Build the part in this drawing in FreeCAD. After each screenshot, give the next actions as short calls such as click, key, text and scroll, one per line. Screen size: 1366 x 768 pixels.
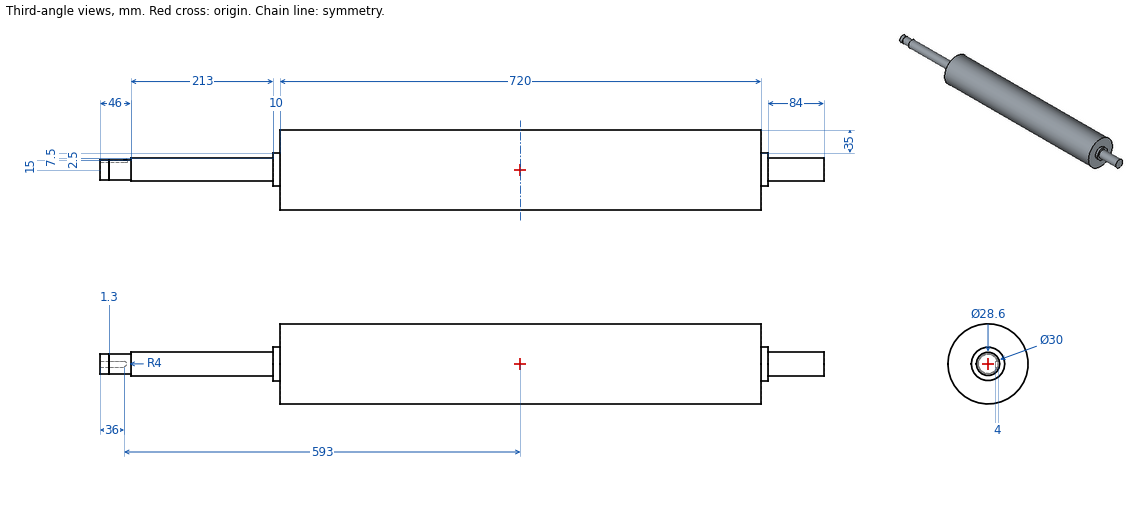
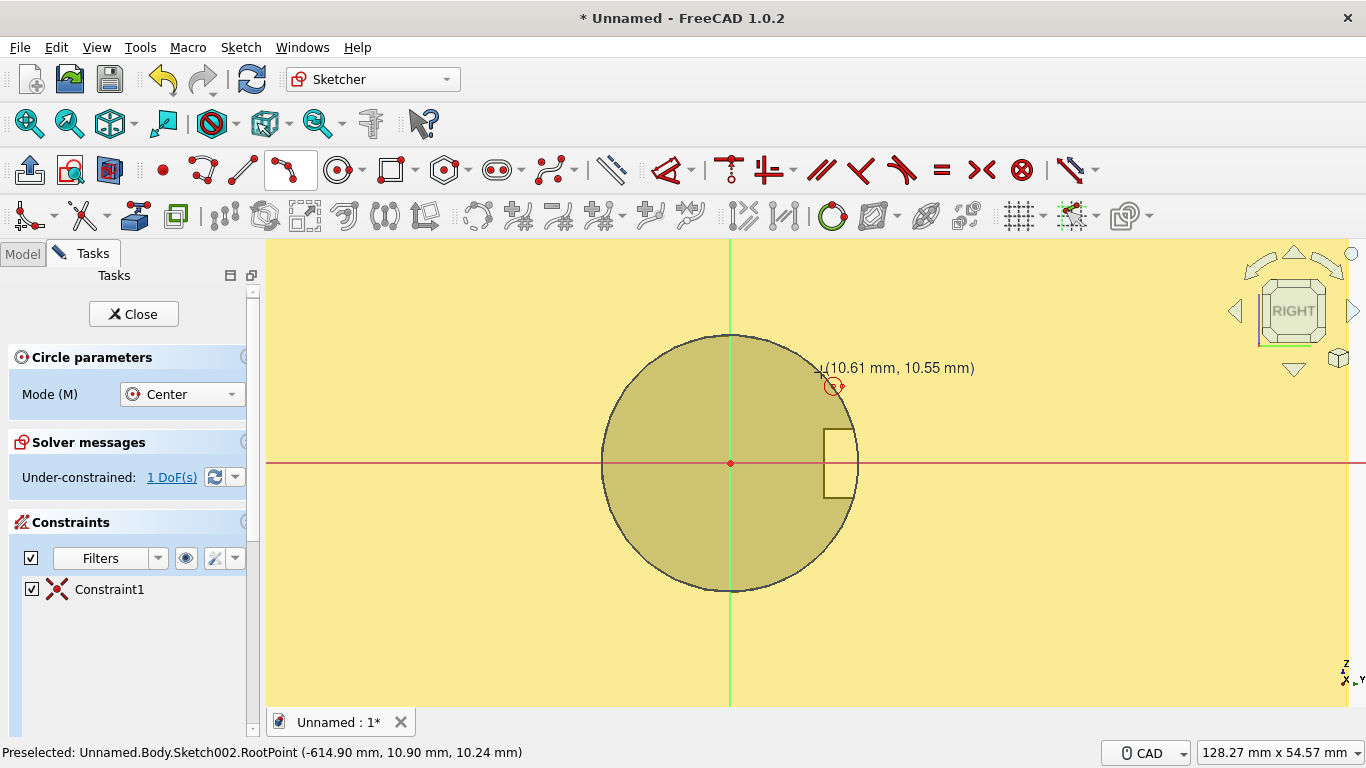
click(730, 463)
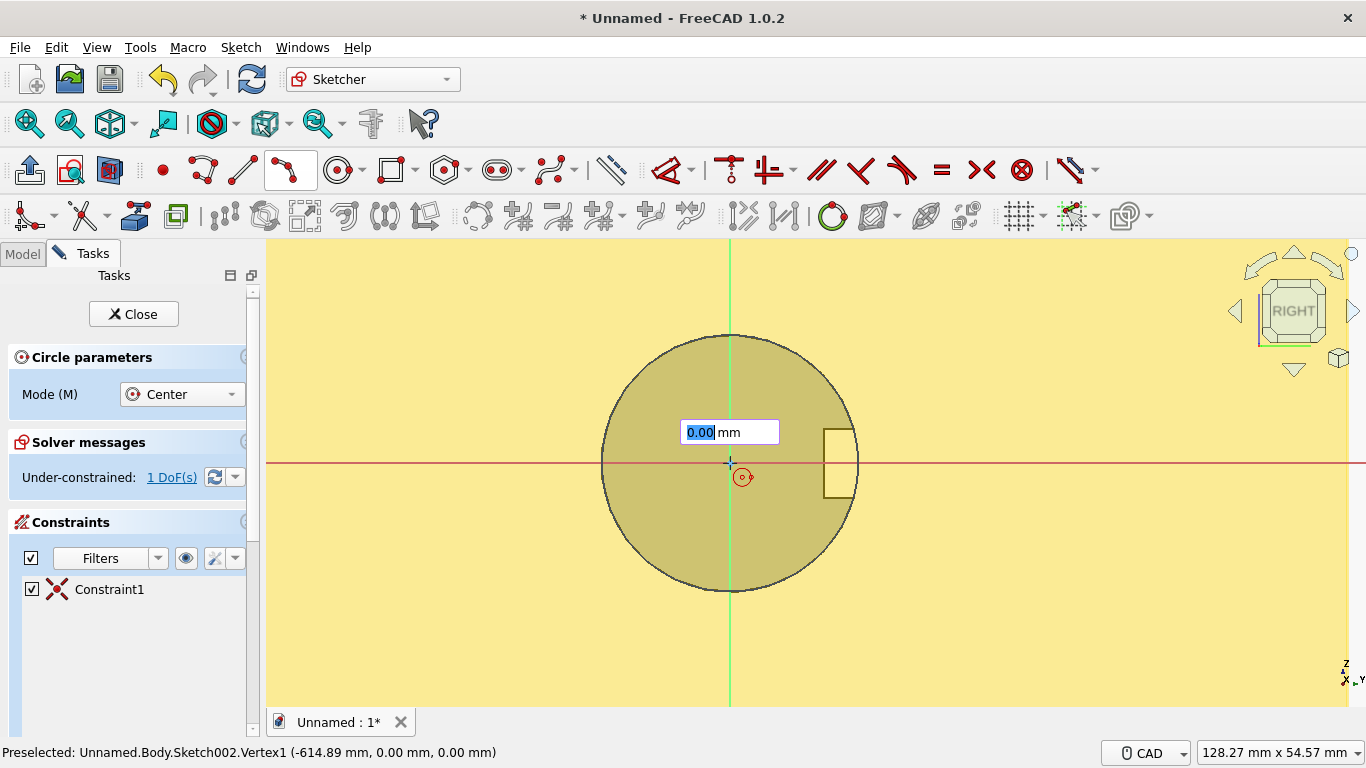
scroll(772, 348, up, 5)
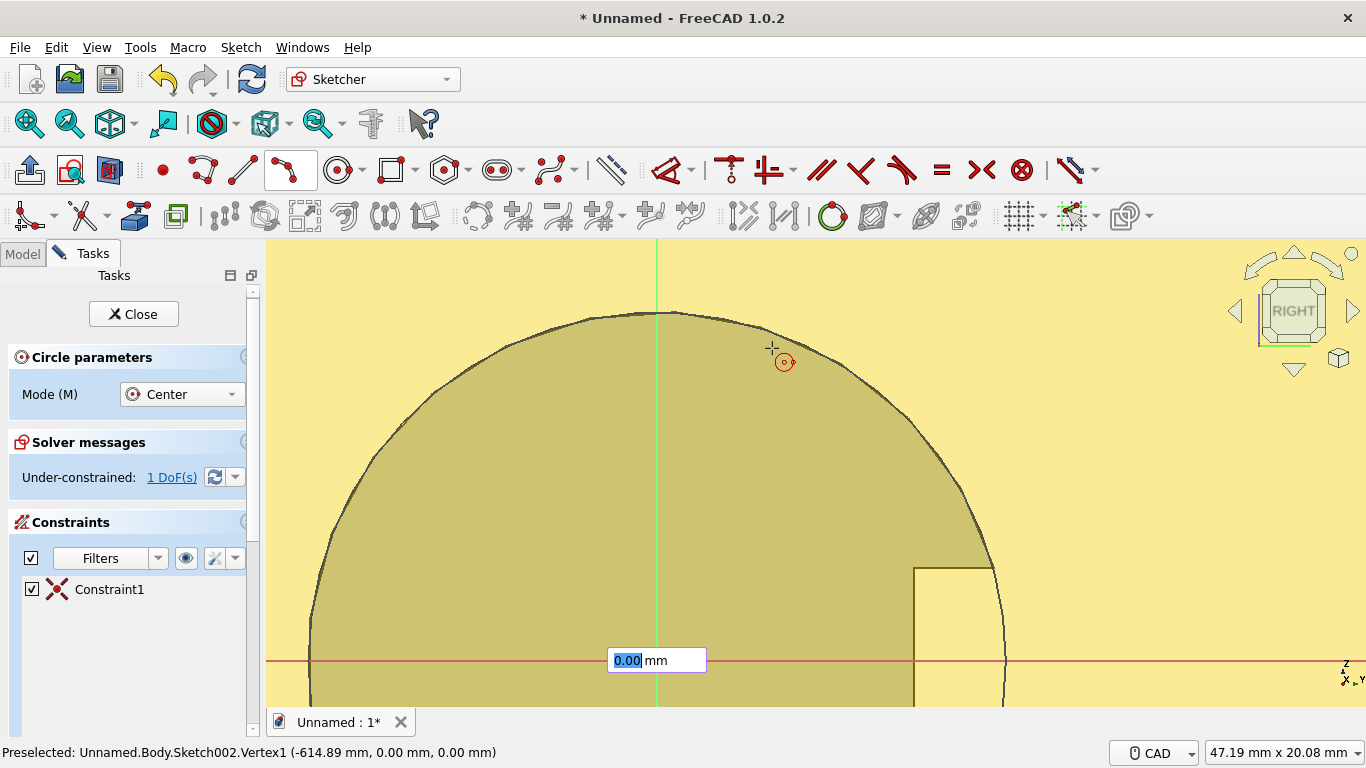
click(771, 348)
key(Escape)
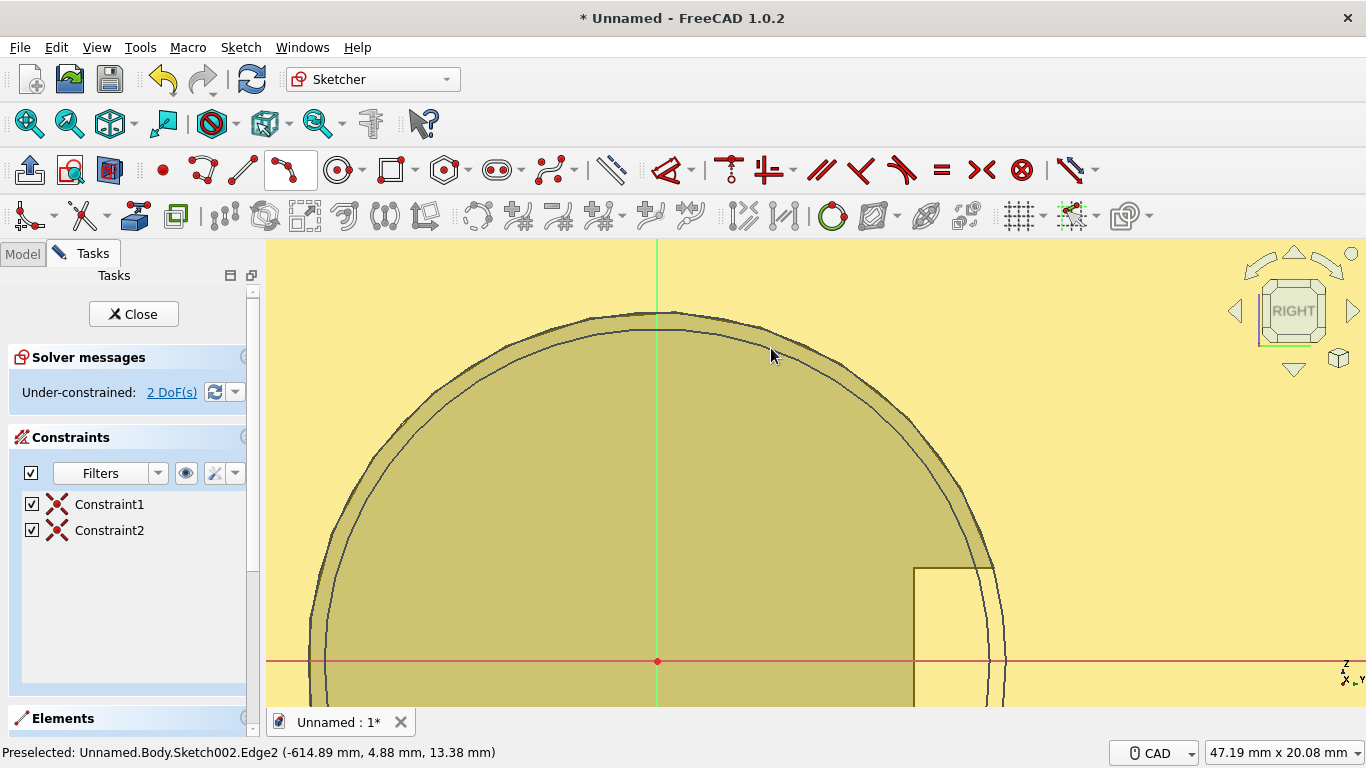
key(d)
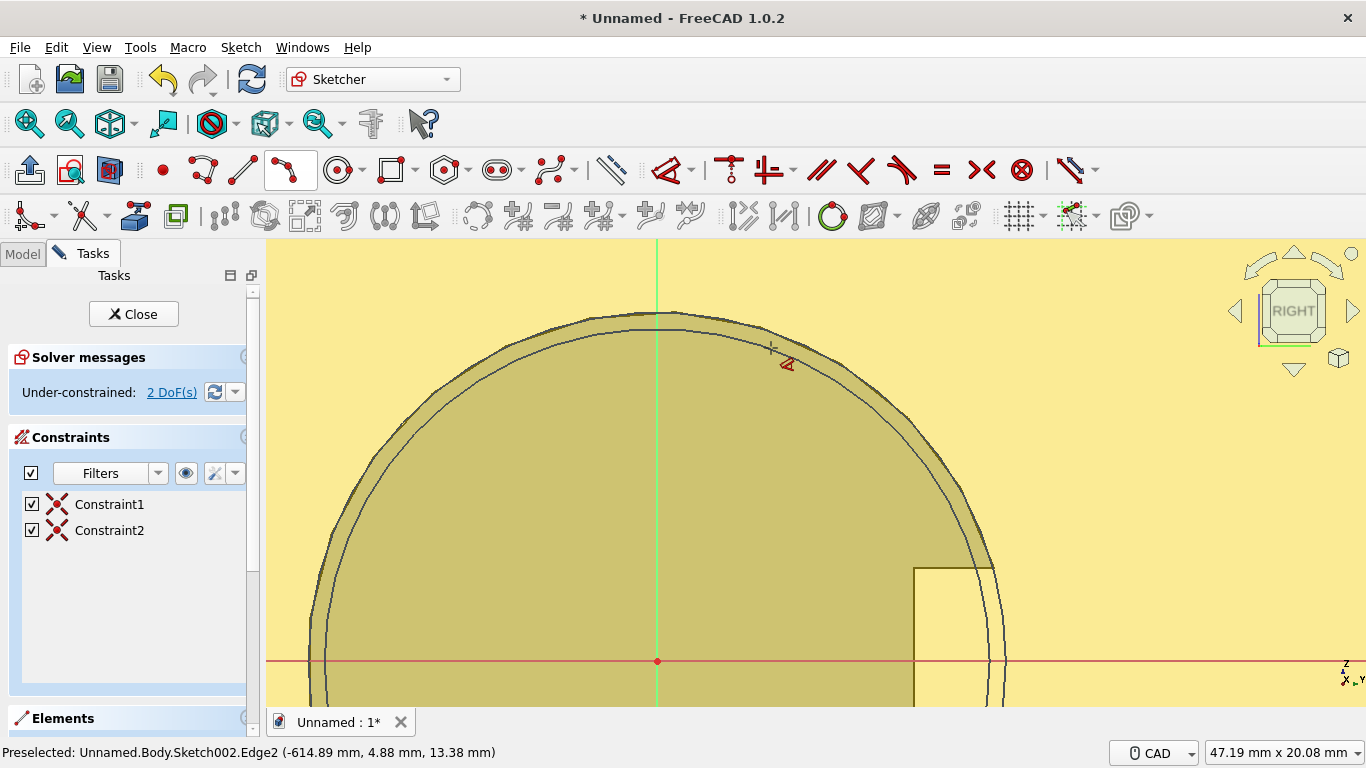
click(903, 414)
click(926, 391)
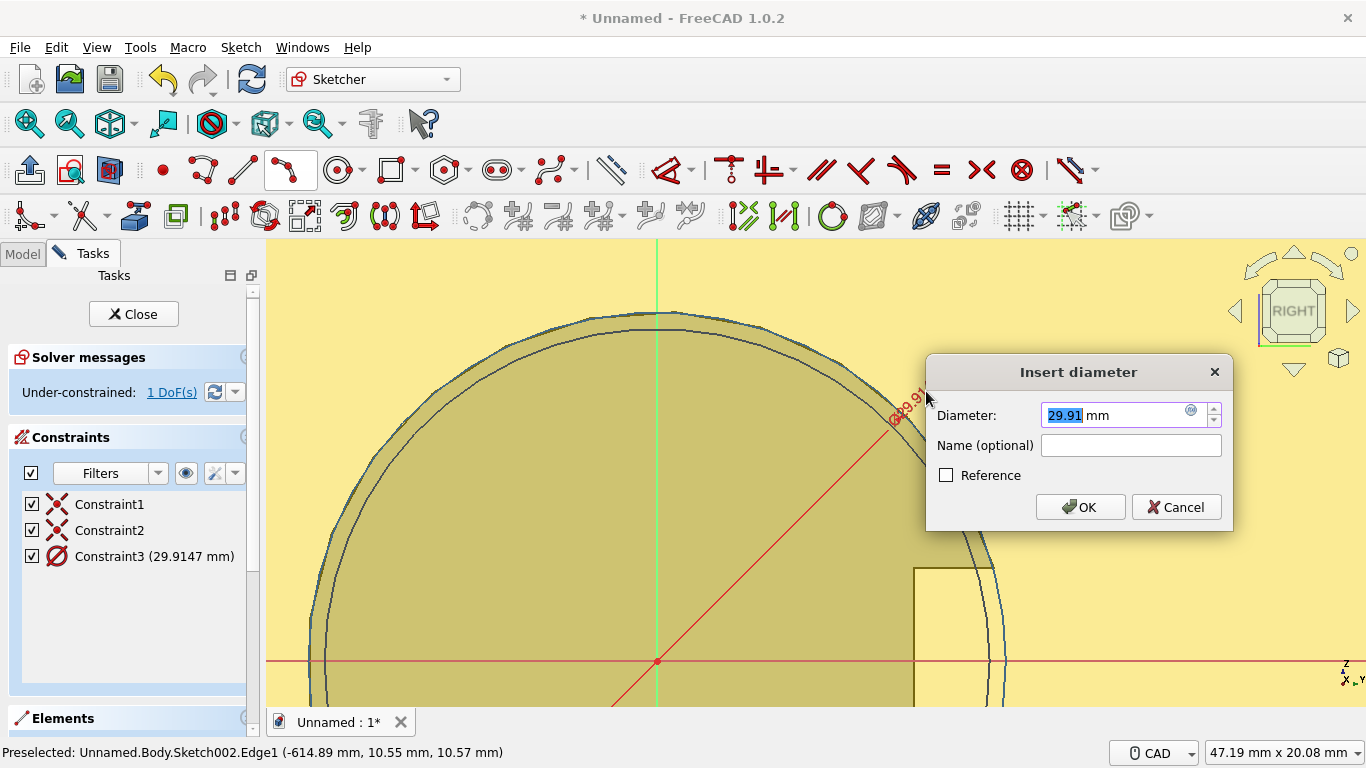
text(30)
key(Return)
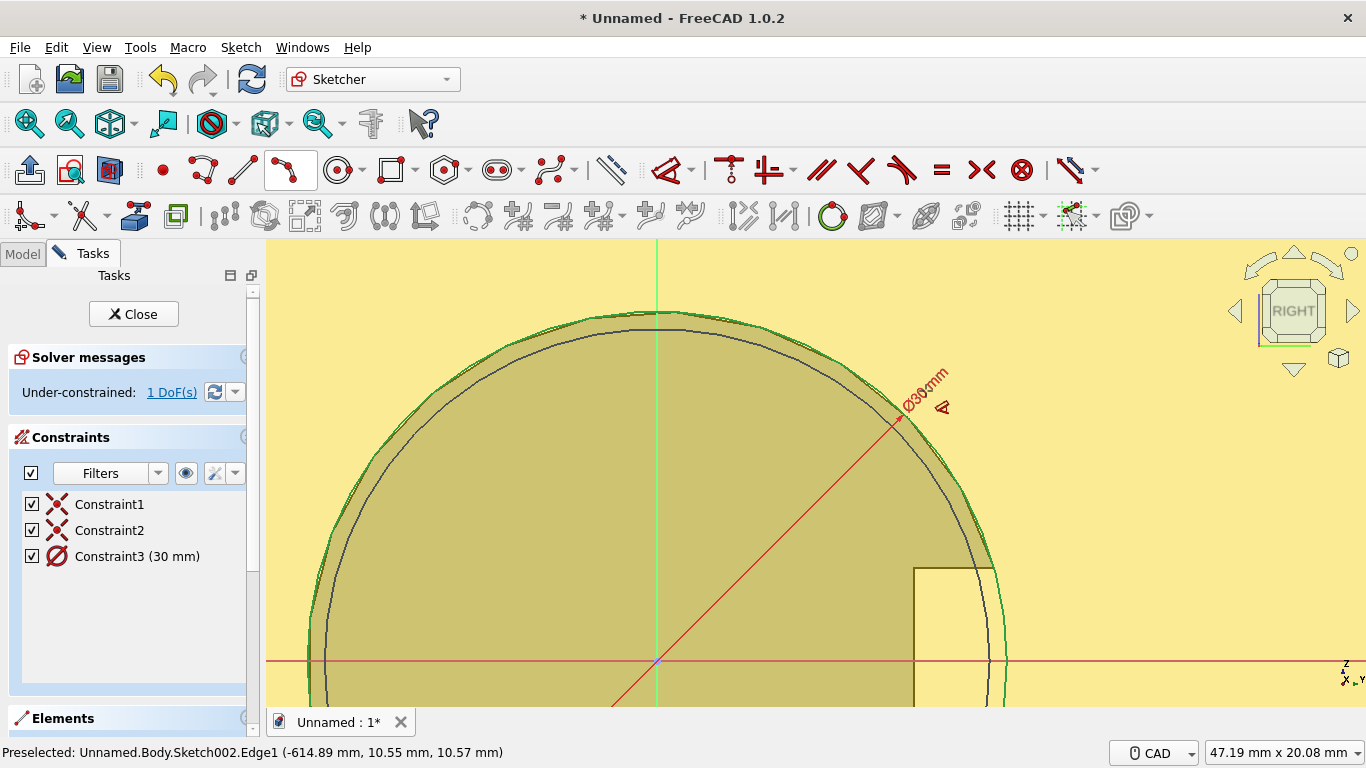
click(892, 426)
click(1007, 558)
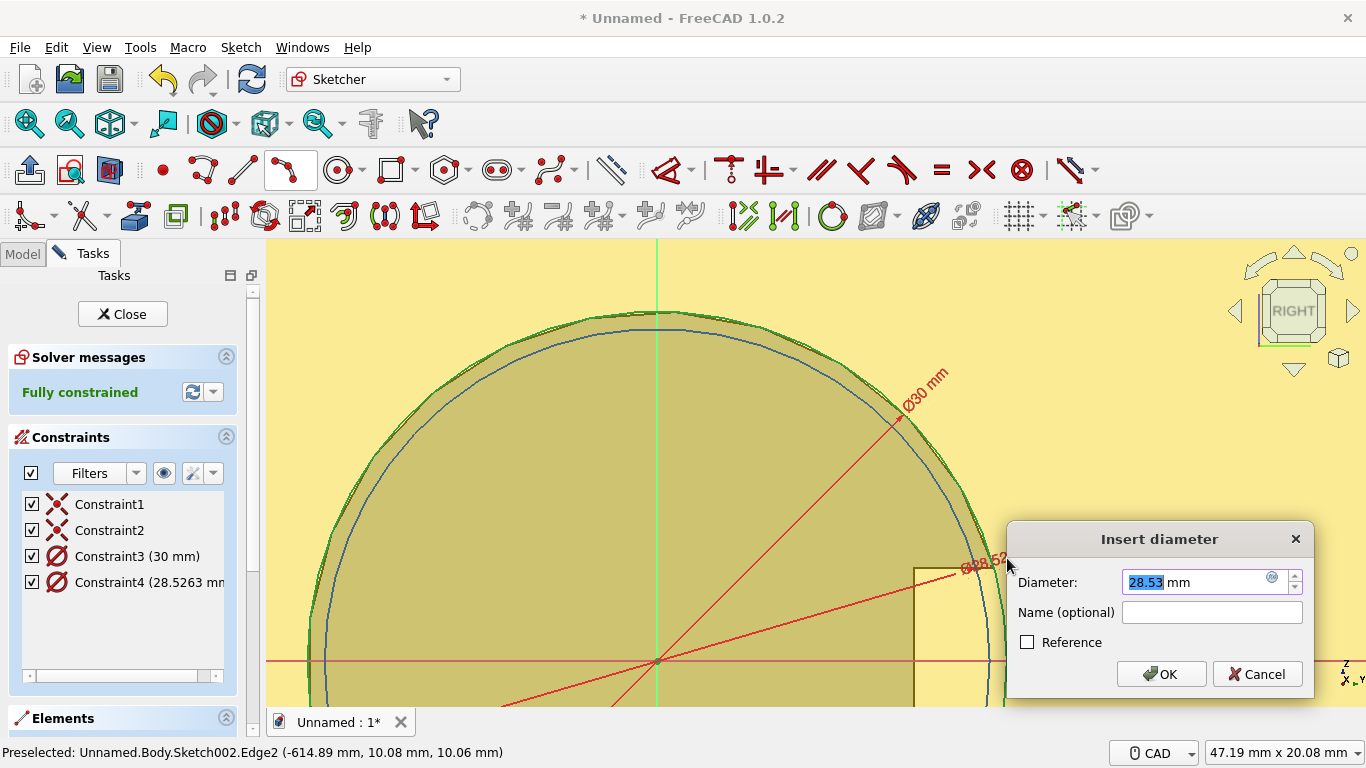
text(28.6)
key(Return)
key(Escape)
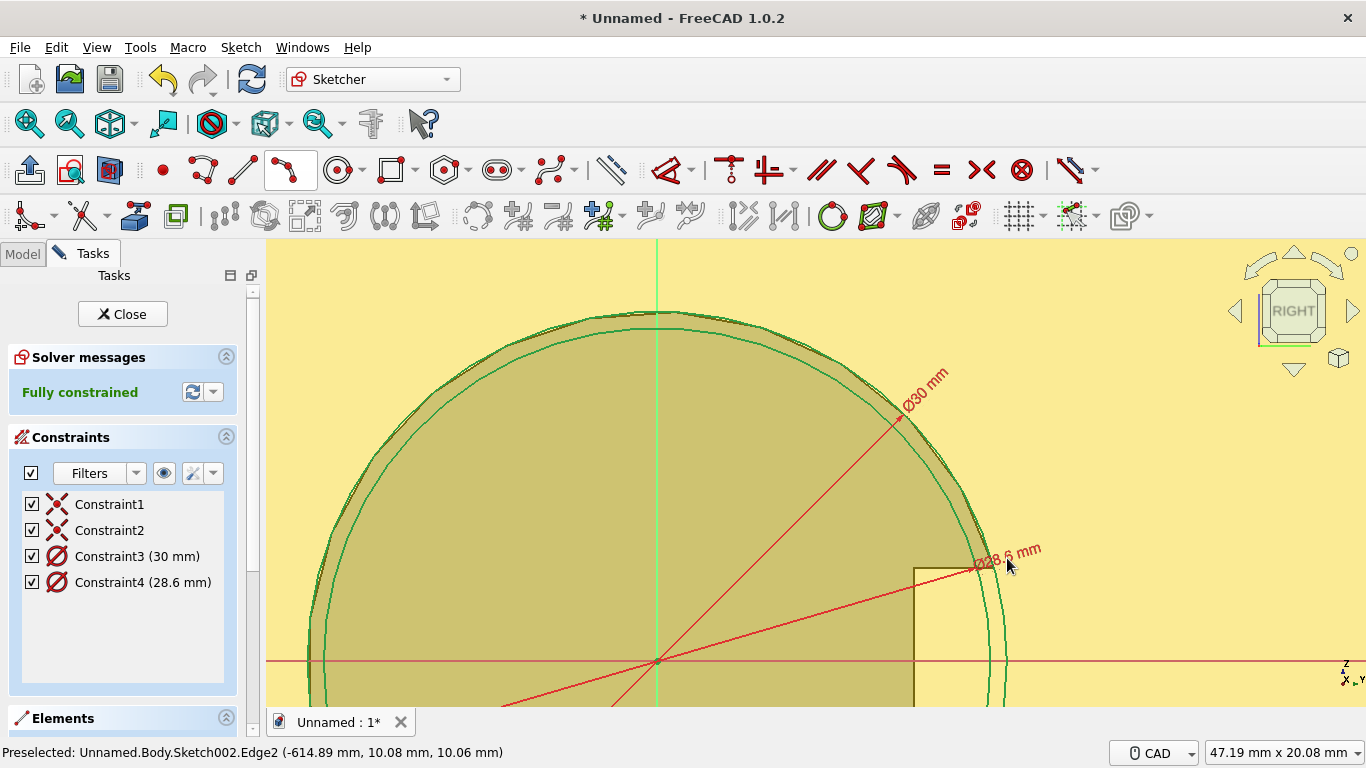
click(123, 314)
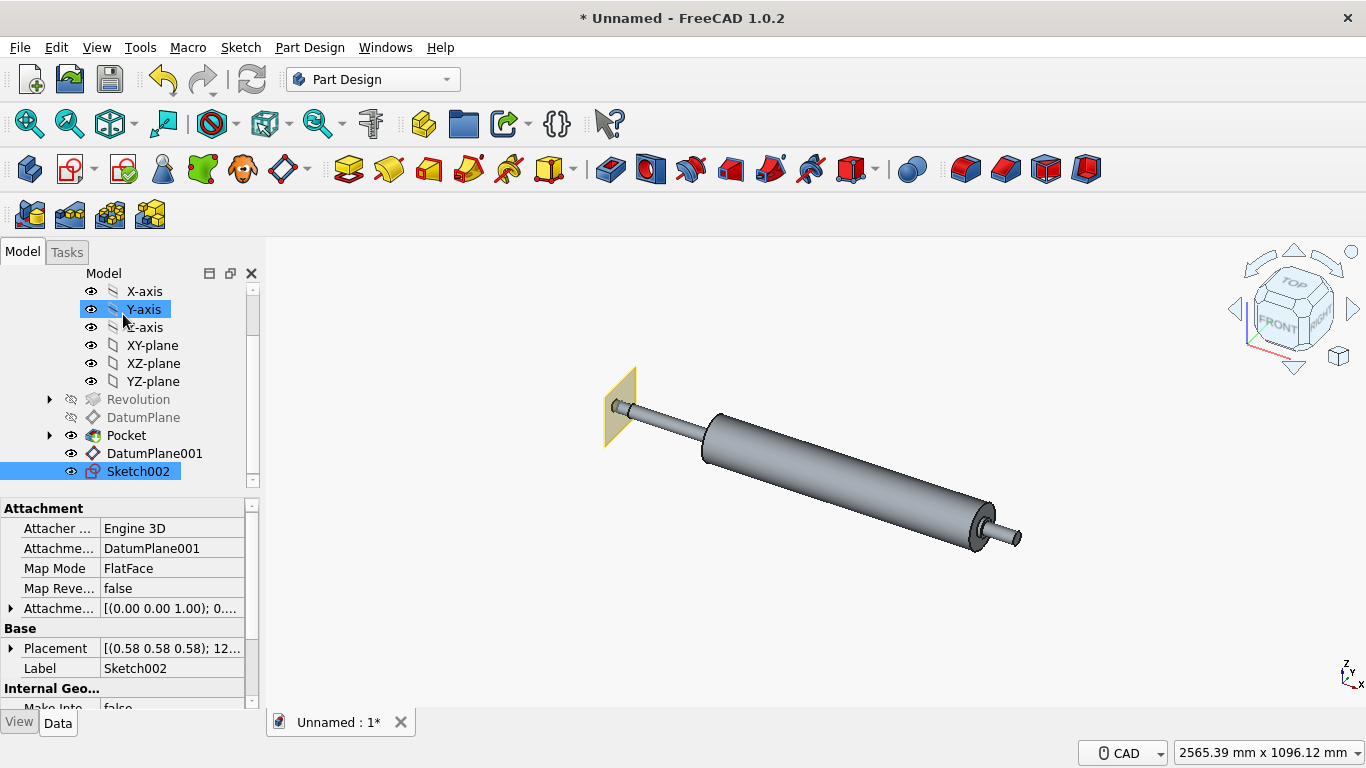
click(612, 170)